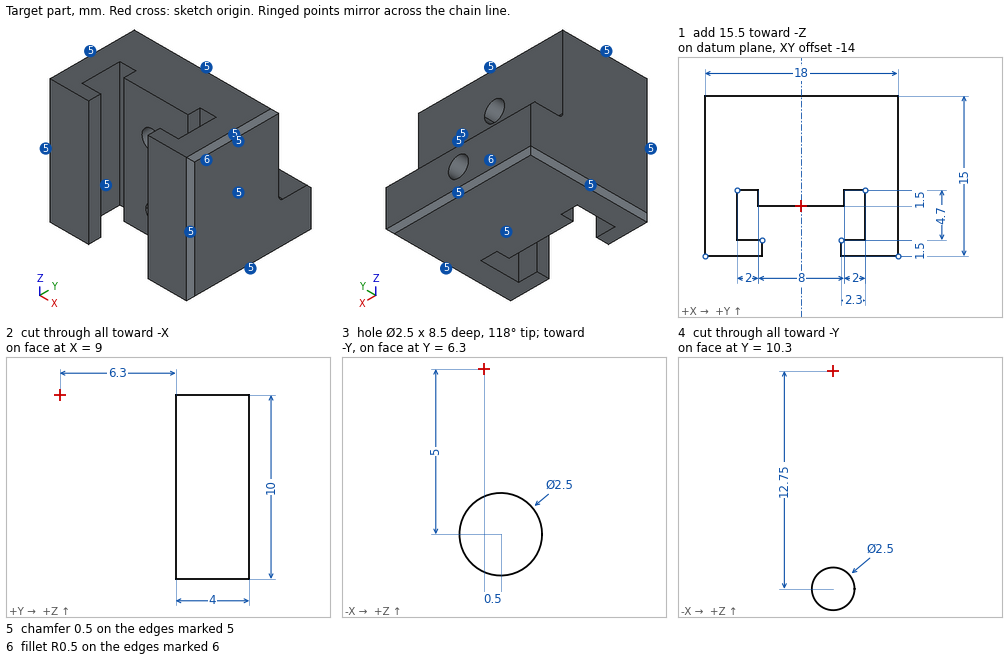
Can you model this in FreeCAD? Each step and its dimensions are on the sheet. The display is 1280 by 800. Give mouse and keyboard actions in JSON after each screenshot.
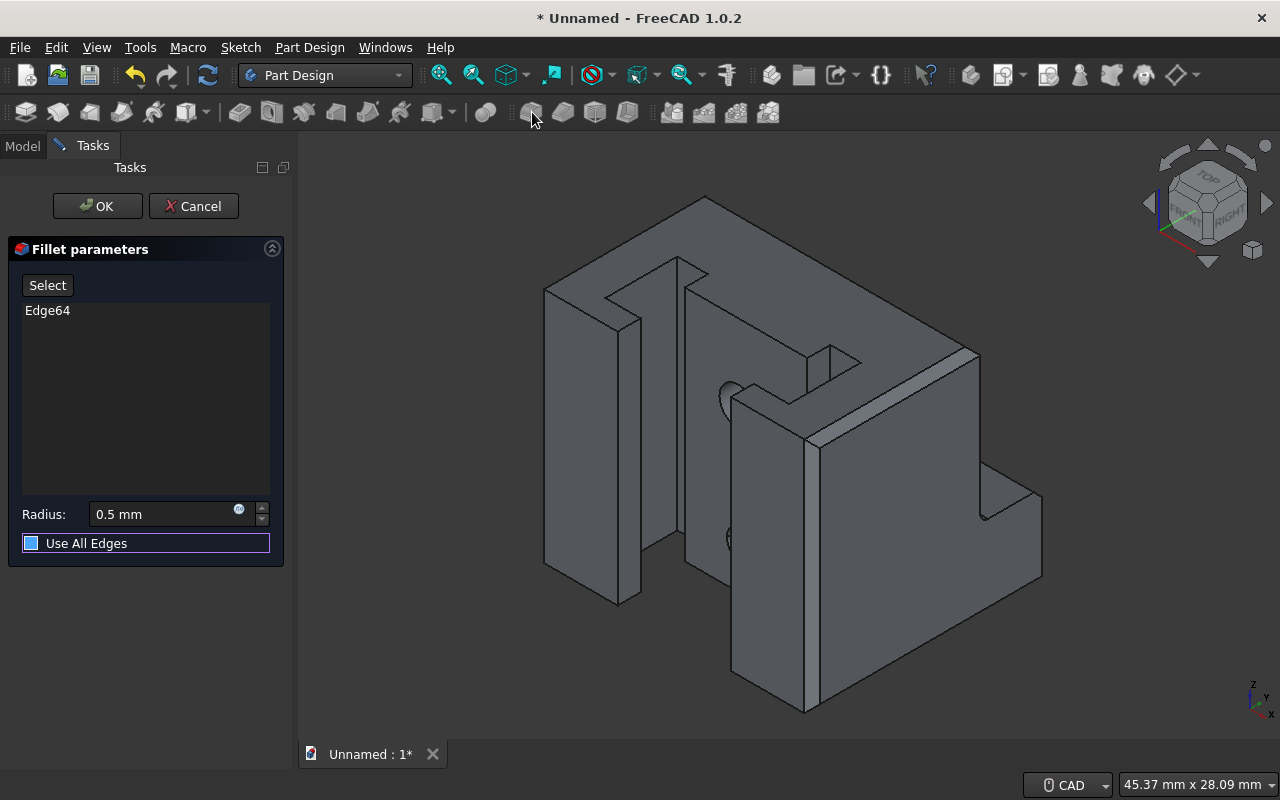
{"action": "left_click", "coordinate": [98, 206]}